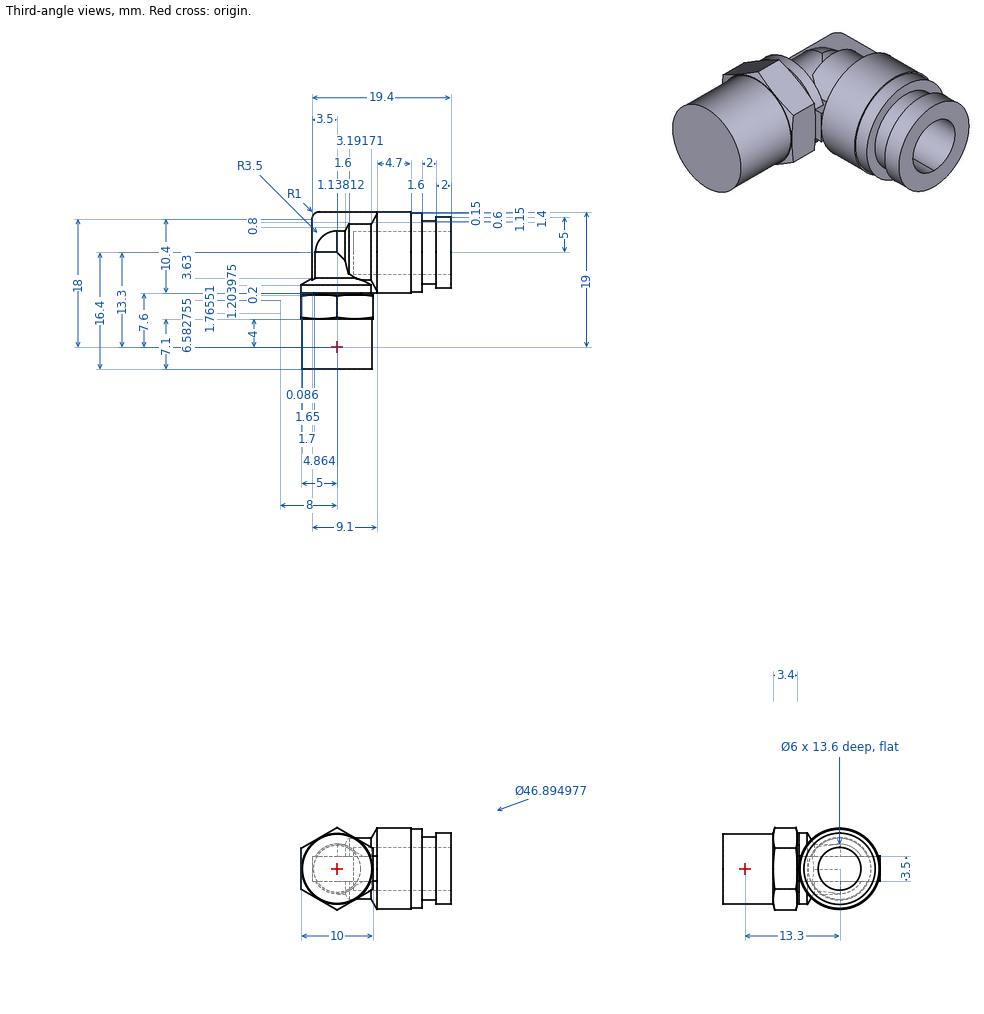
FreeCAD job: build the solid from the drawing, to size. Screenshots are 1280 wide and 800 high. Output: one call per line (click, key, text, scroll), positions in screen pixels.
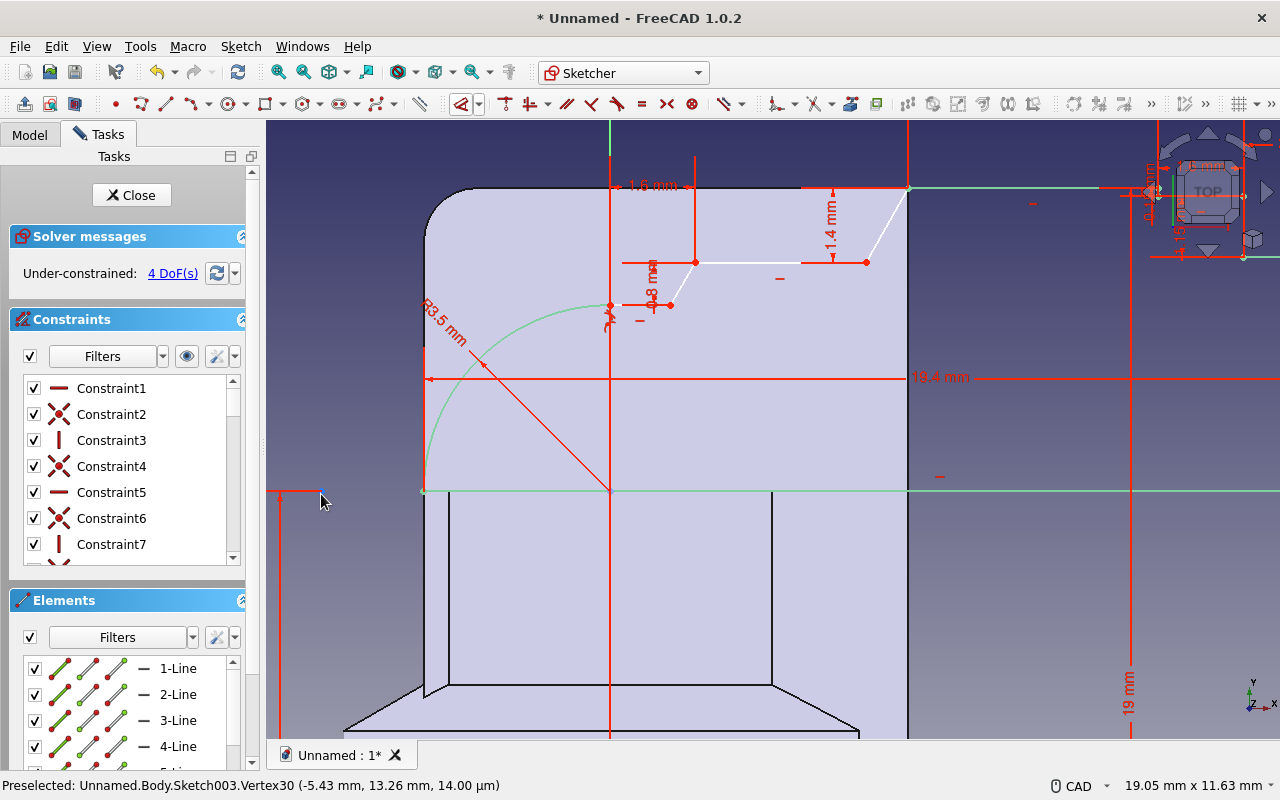
click(815, 263)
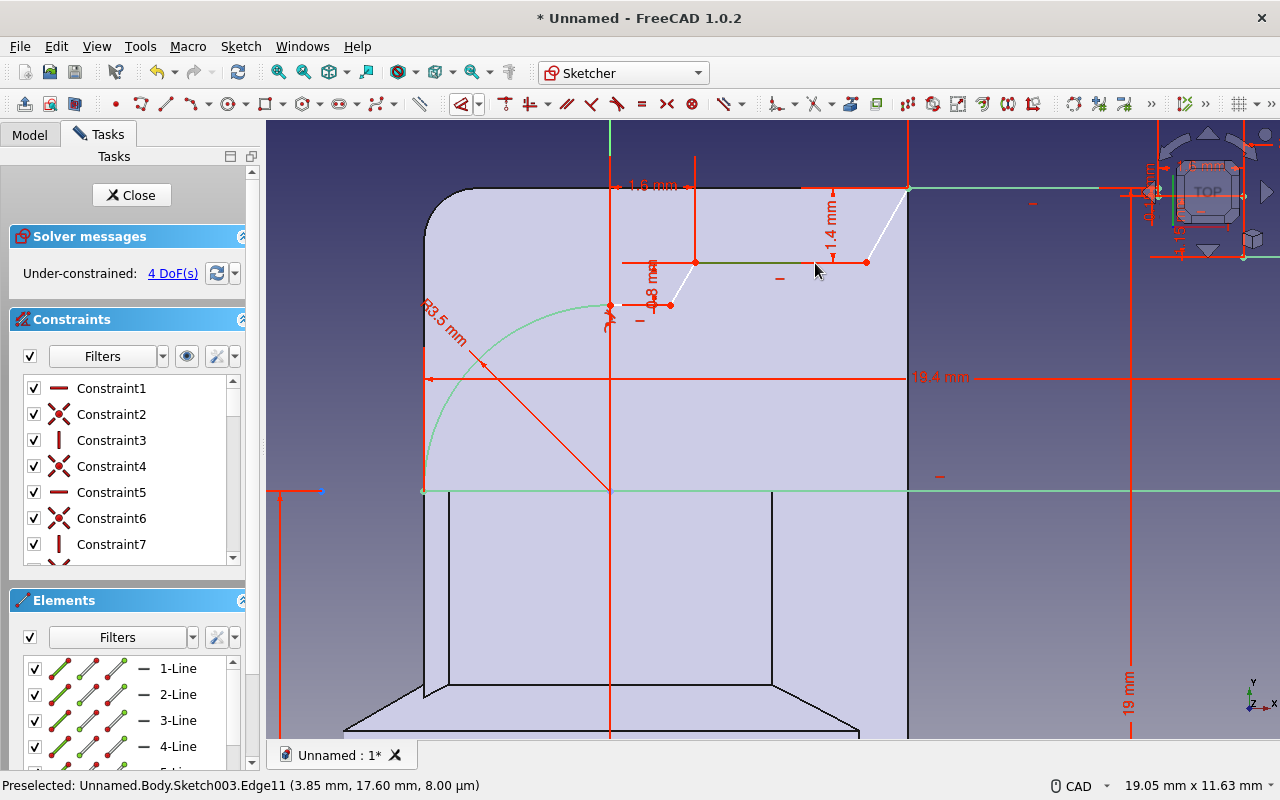
key(l)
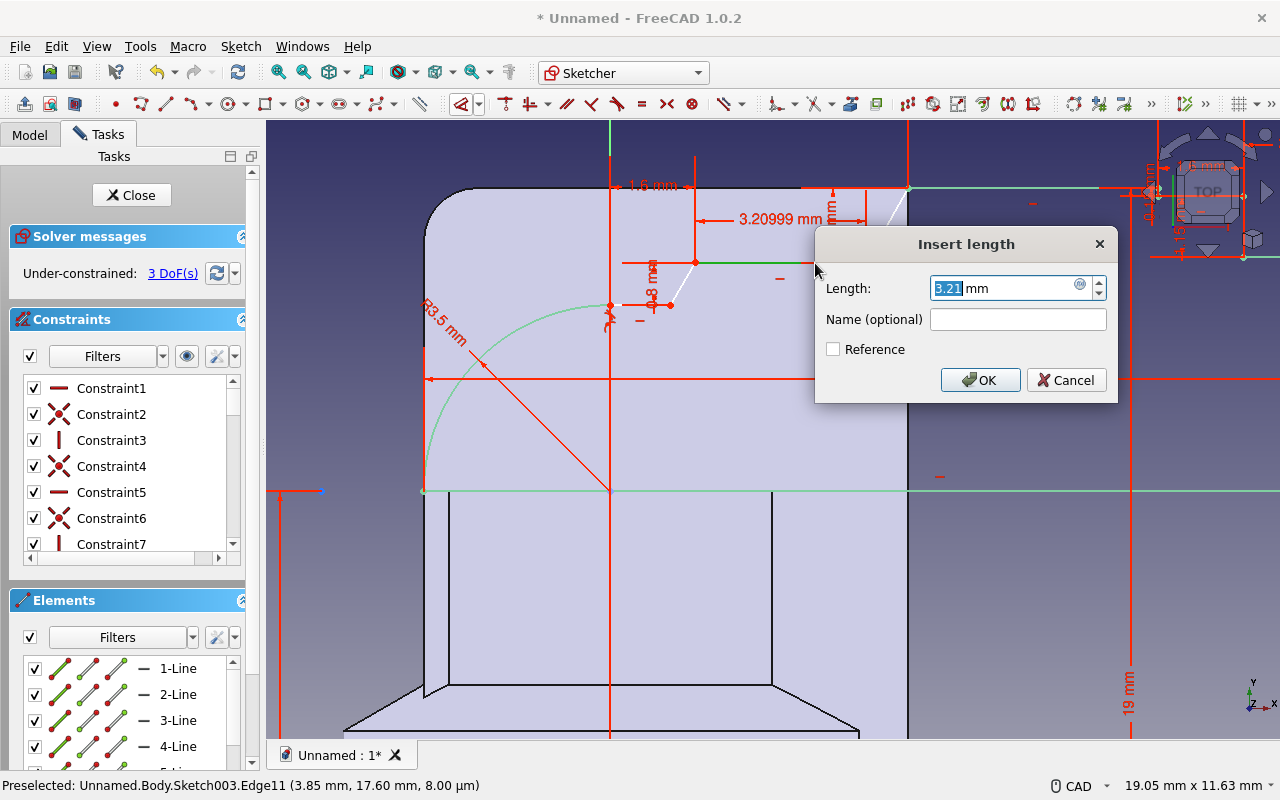
text(3.19171)
key(Return)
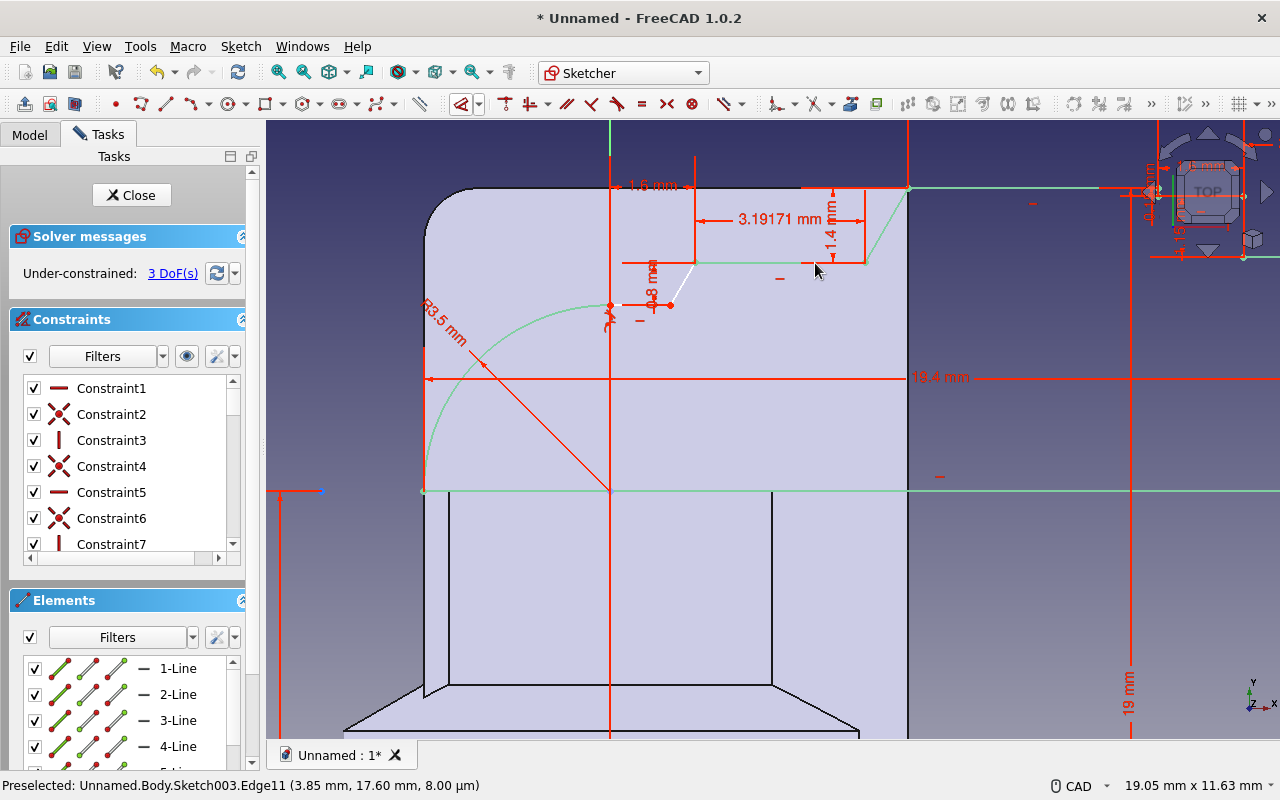
click(628, 305)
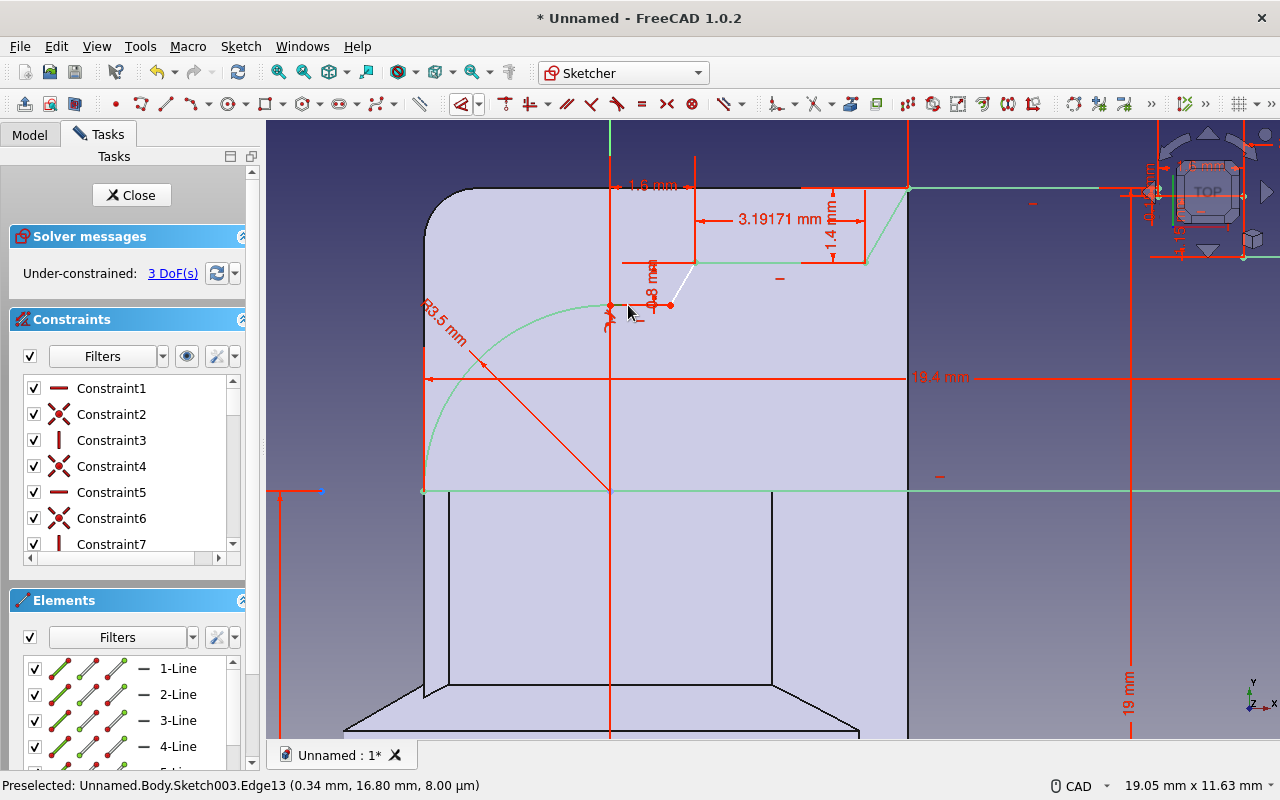
key(l)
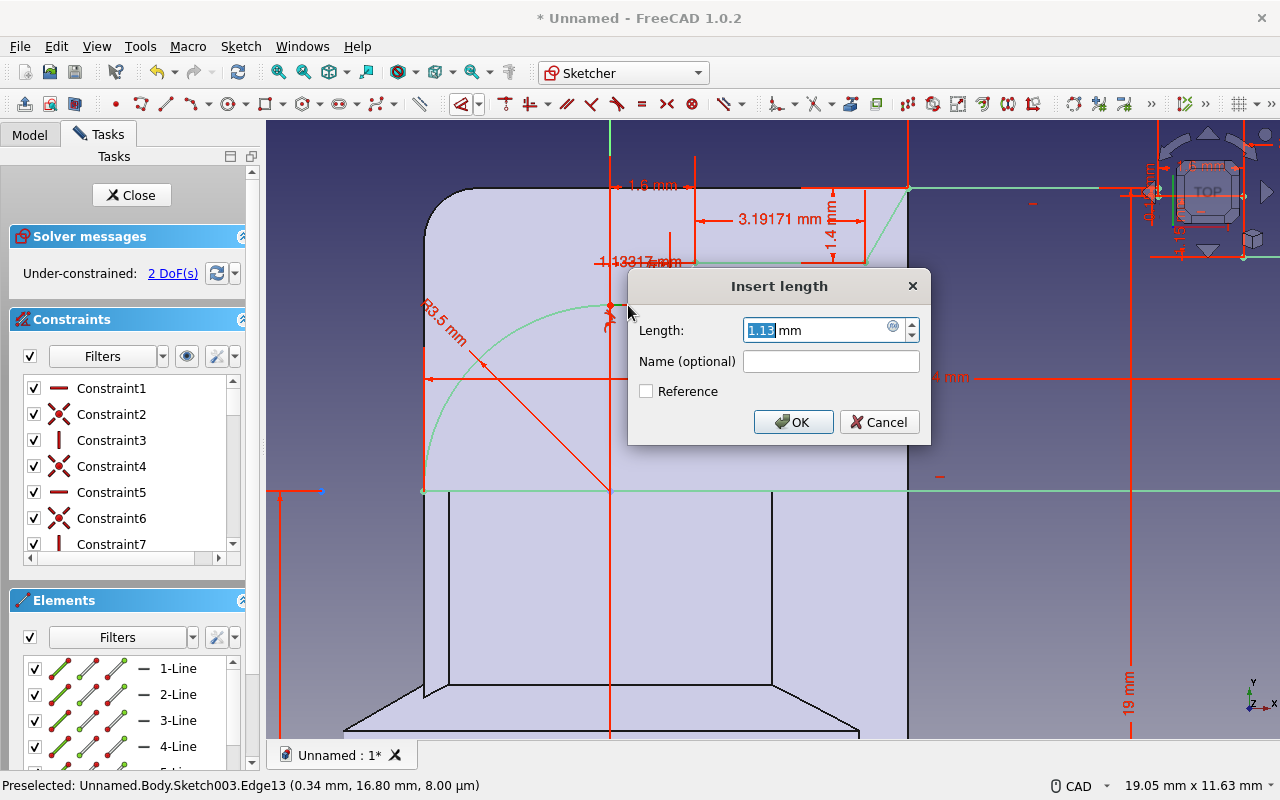
text(1.13812)
key(Return)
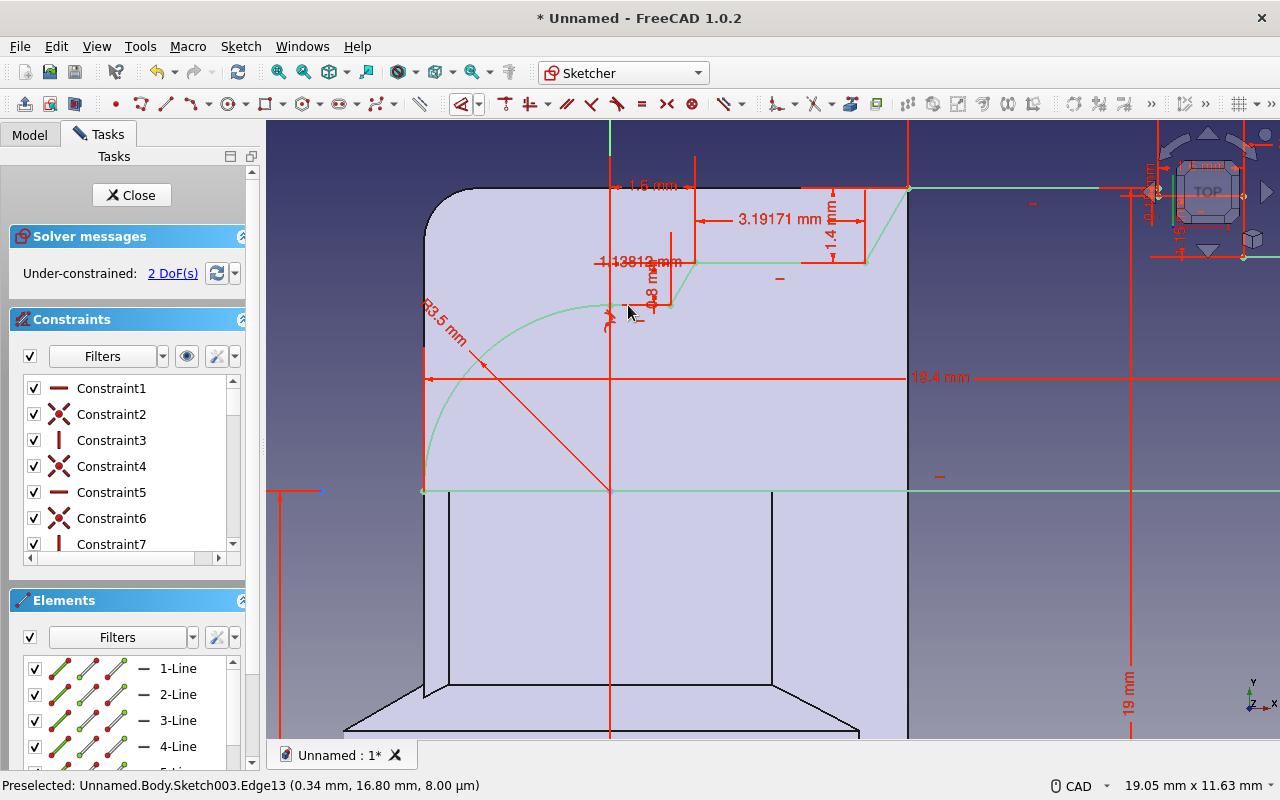
click(132, 195)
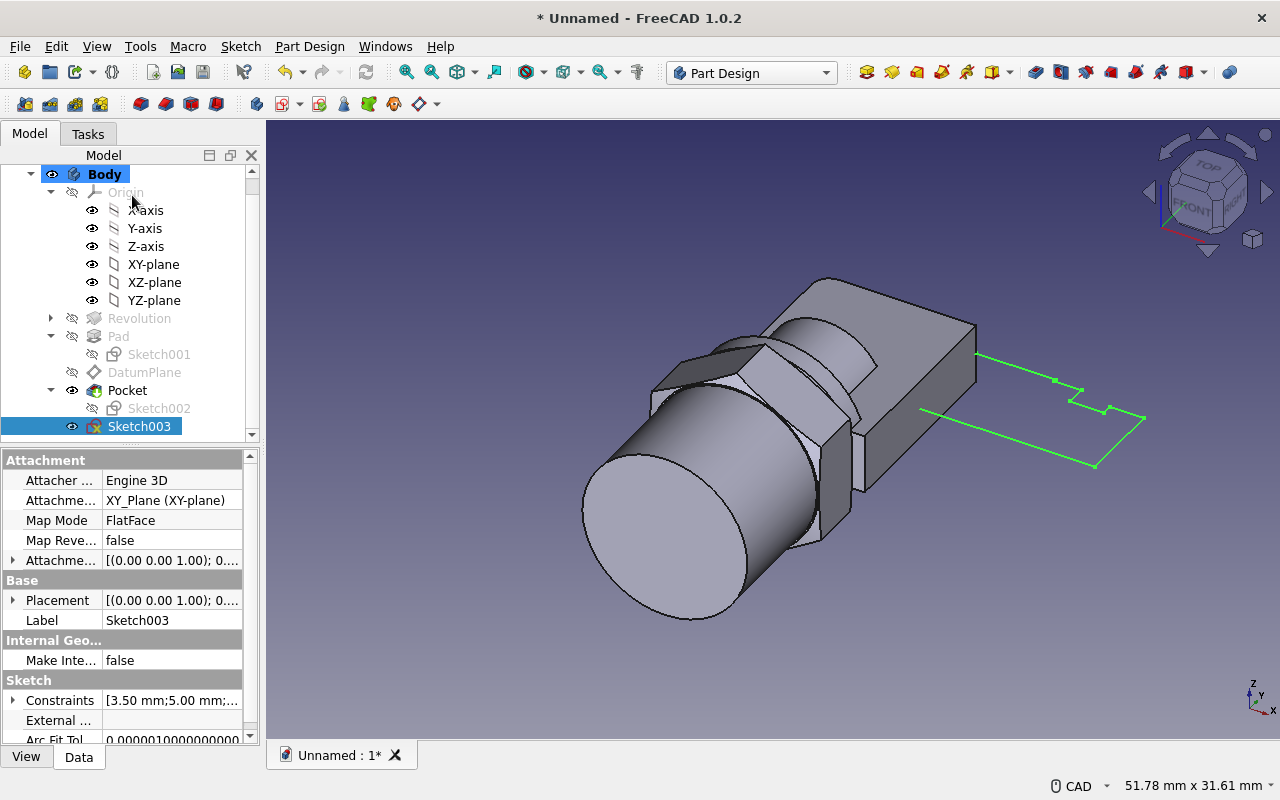
click(892, 72)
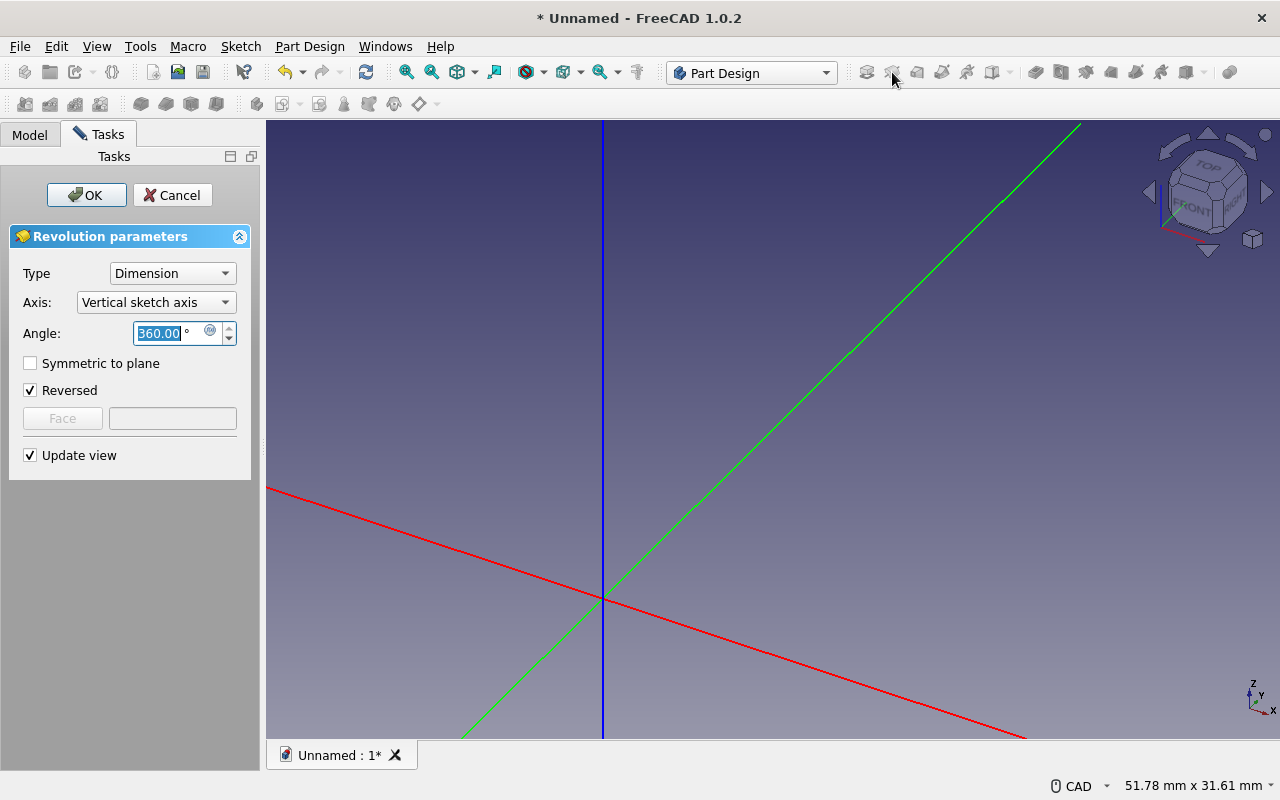
click(157, 302)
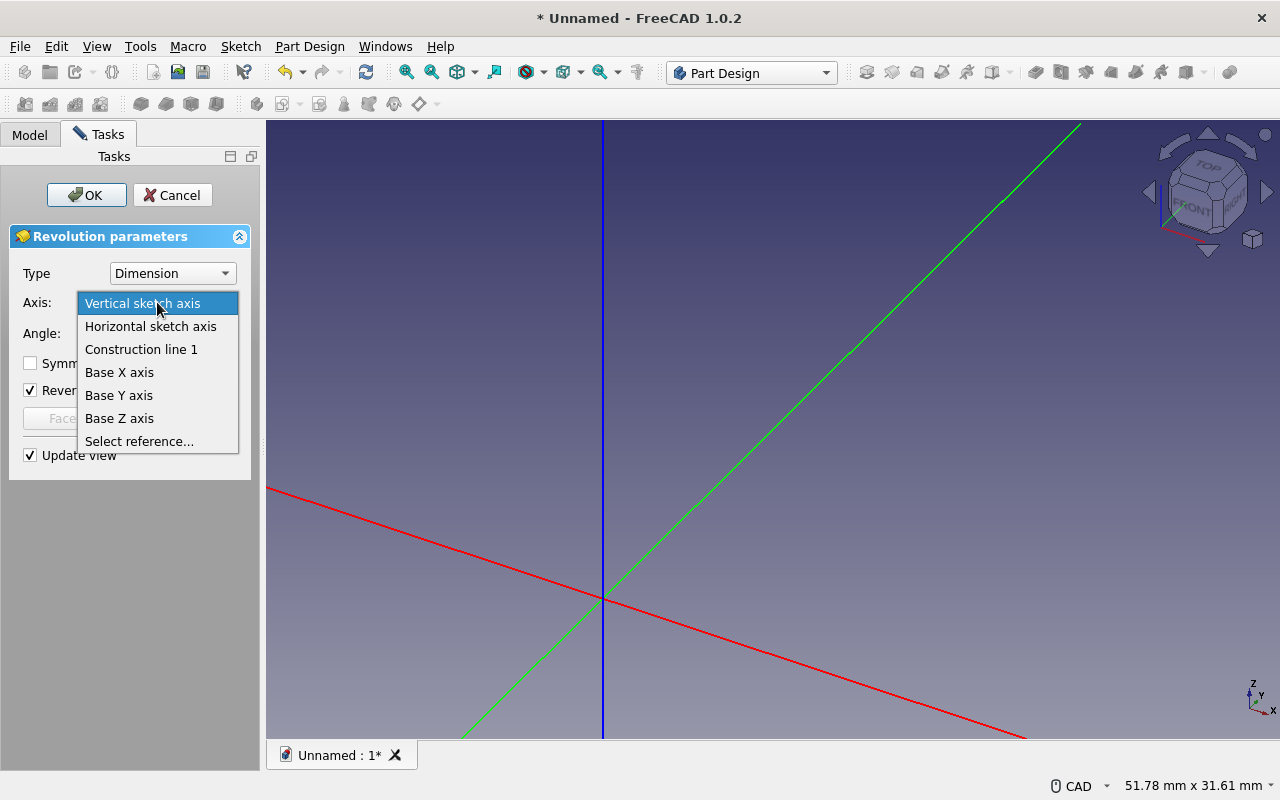
click(156, 350)